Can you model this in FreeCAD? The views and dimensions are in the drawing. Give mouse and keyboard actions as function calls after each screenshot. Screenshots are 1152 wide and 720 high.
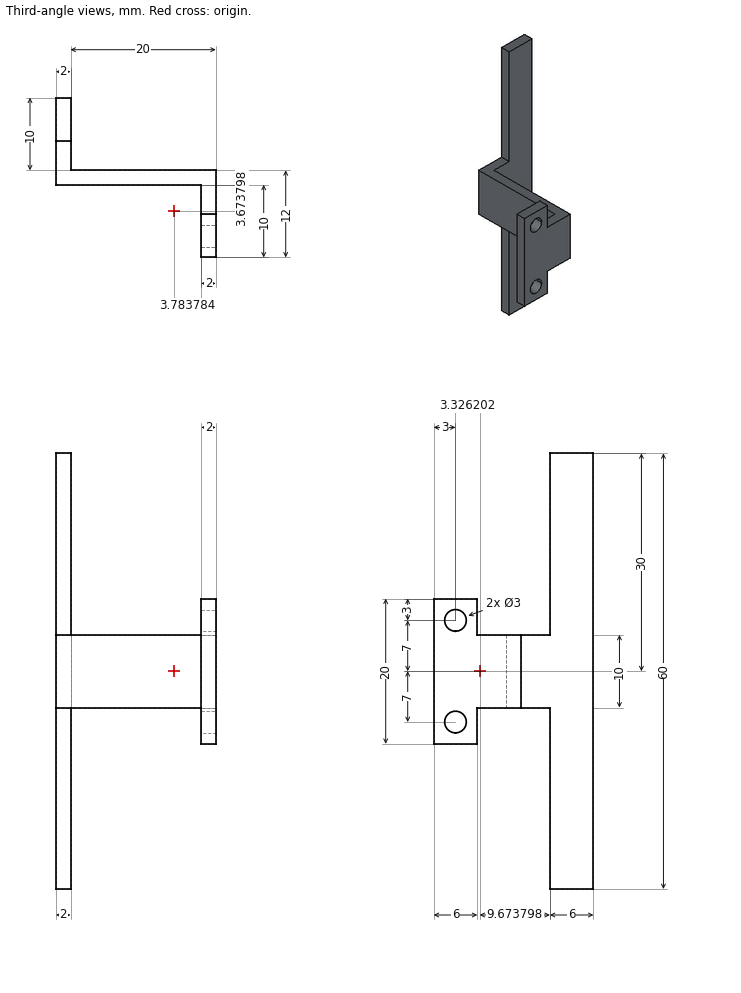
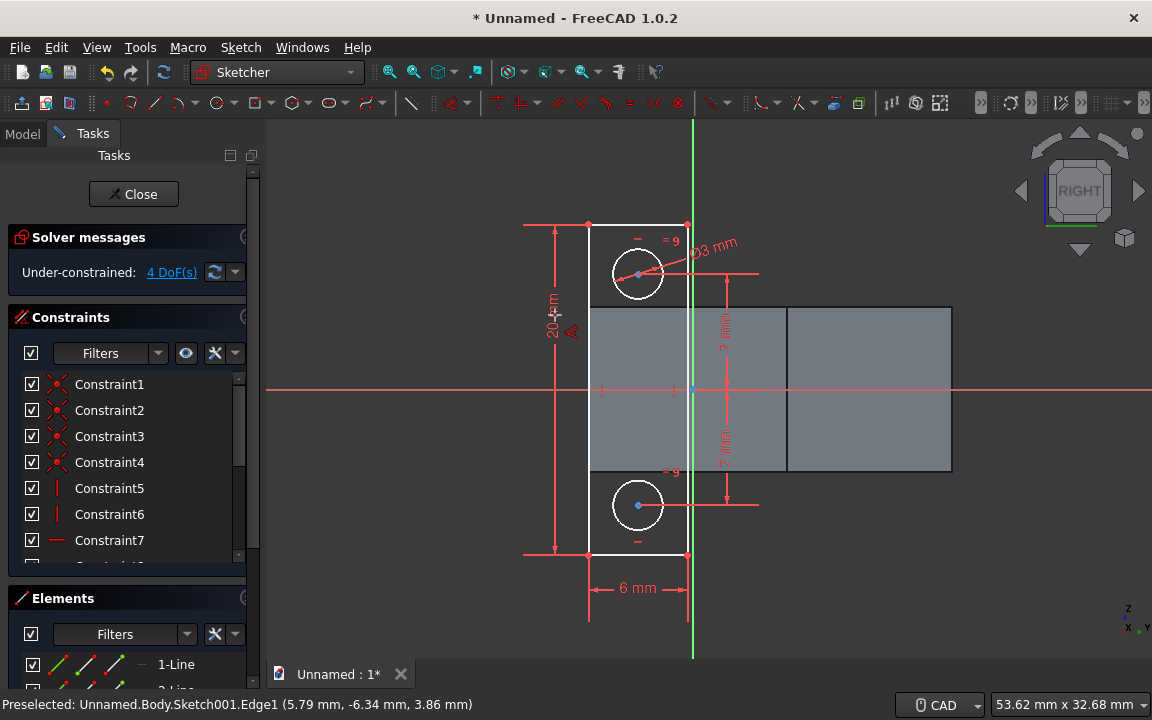
click(589, 225)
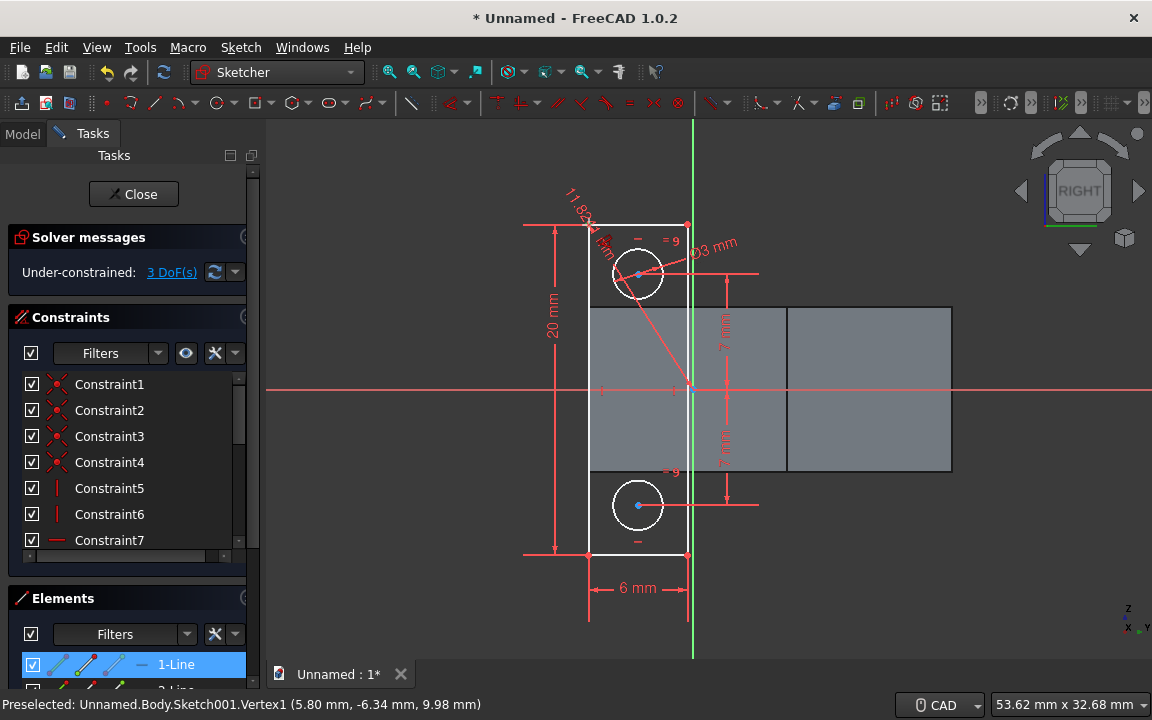
click(638, 274)
click(613, 191)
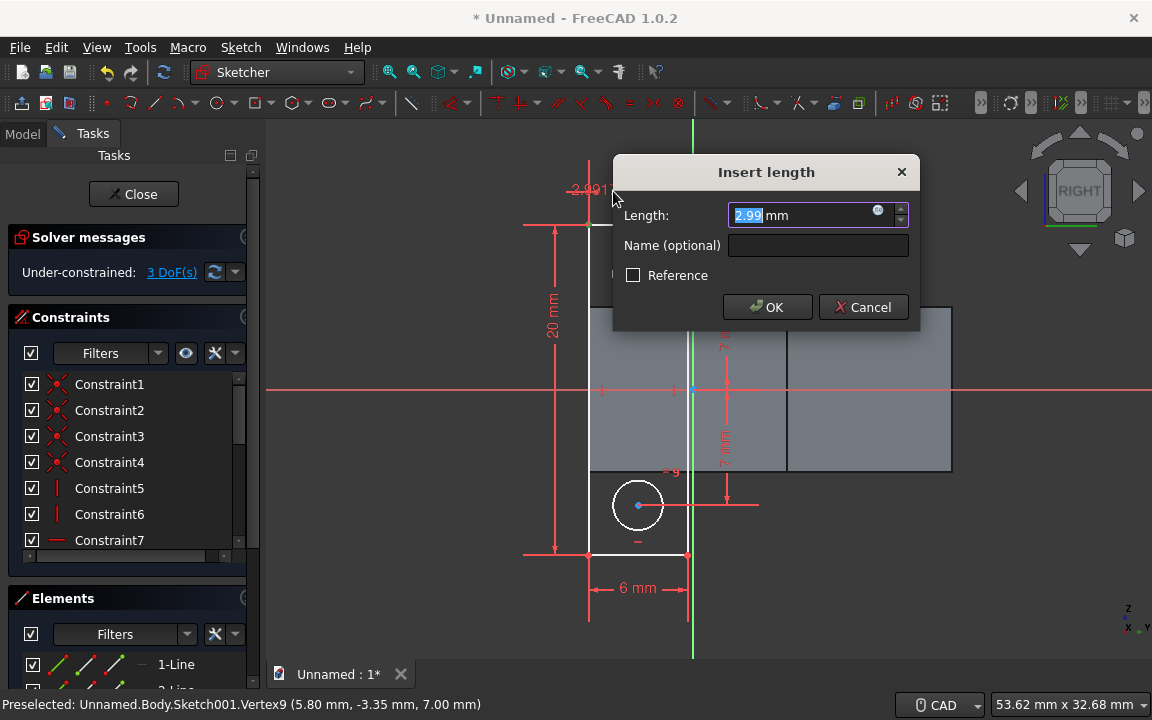
text(3)
key(Return)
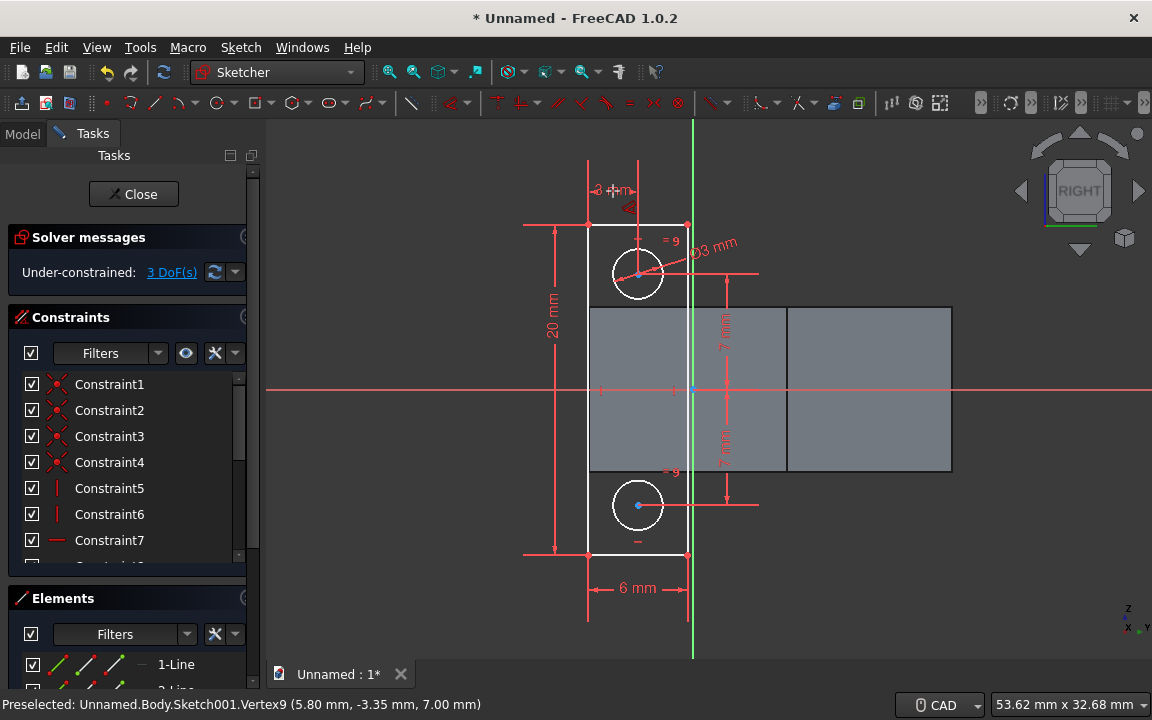
click(588, 225)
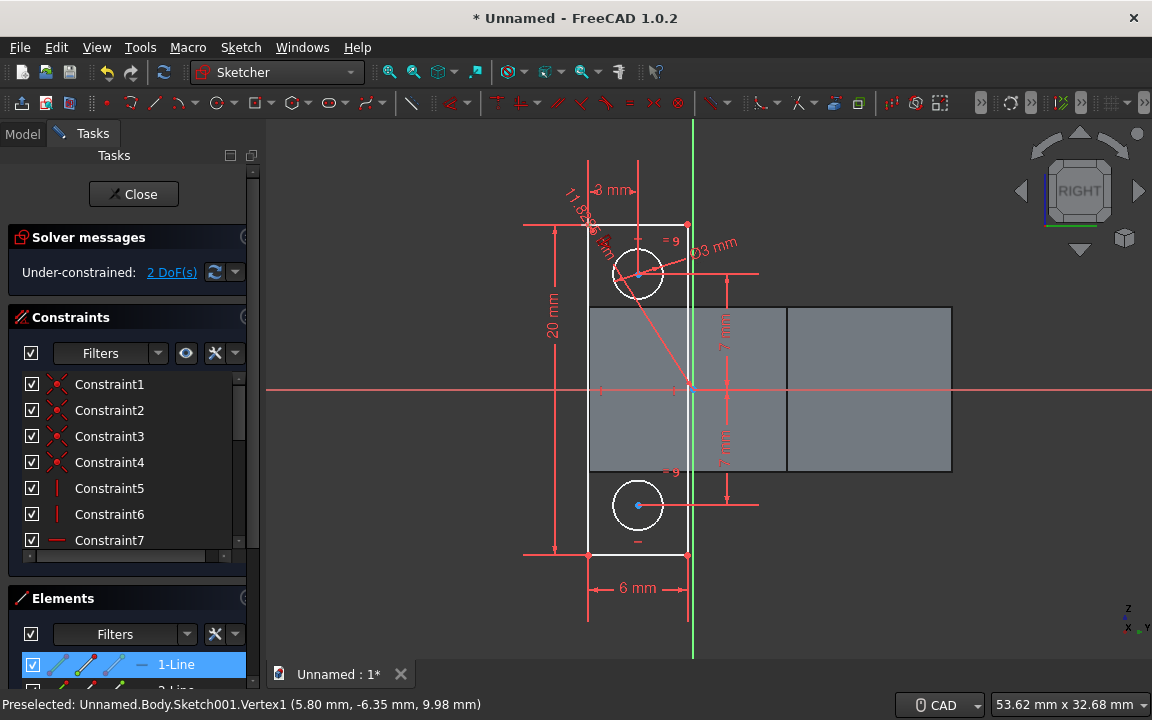
click(638, 274)
click(554, 249)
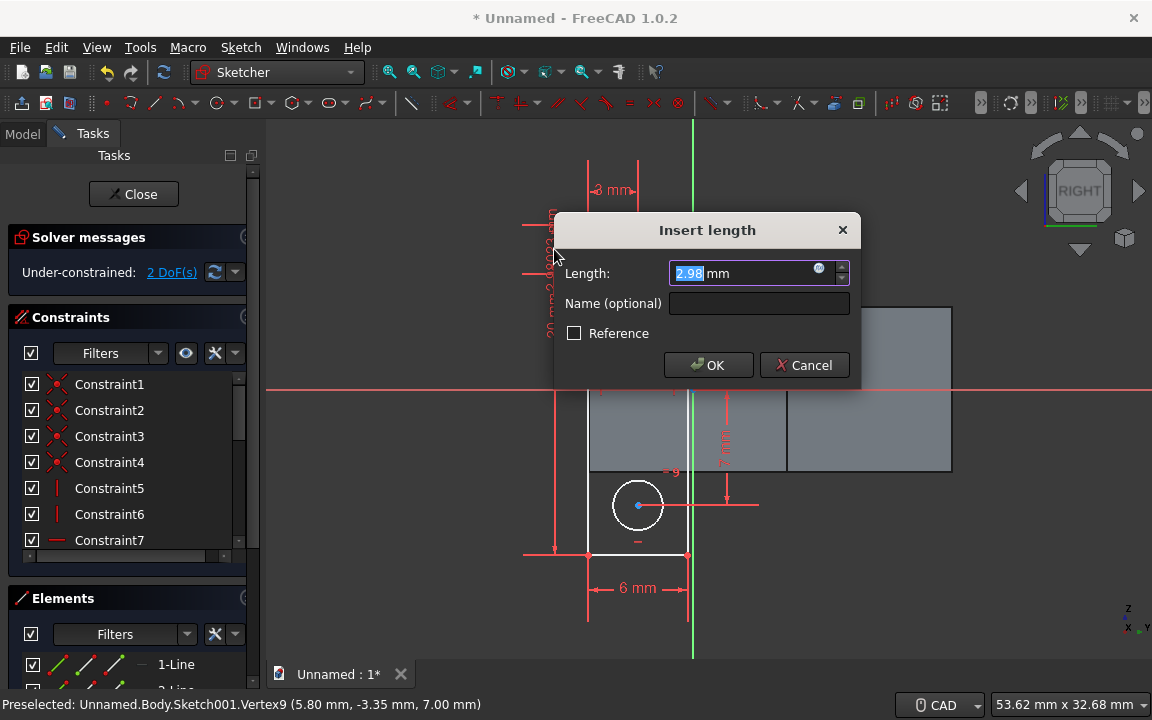
text(3)
key(Return)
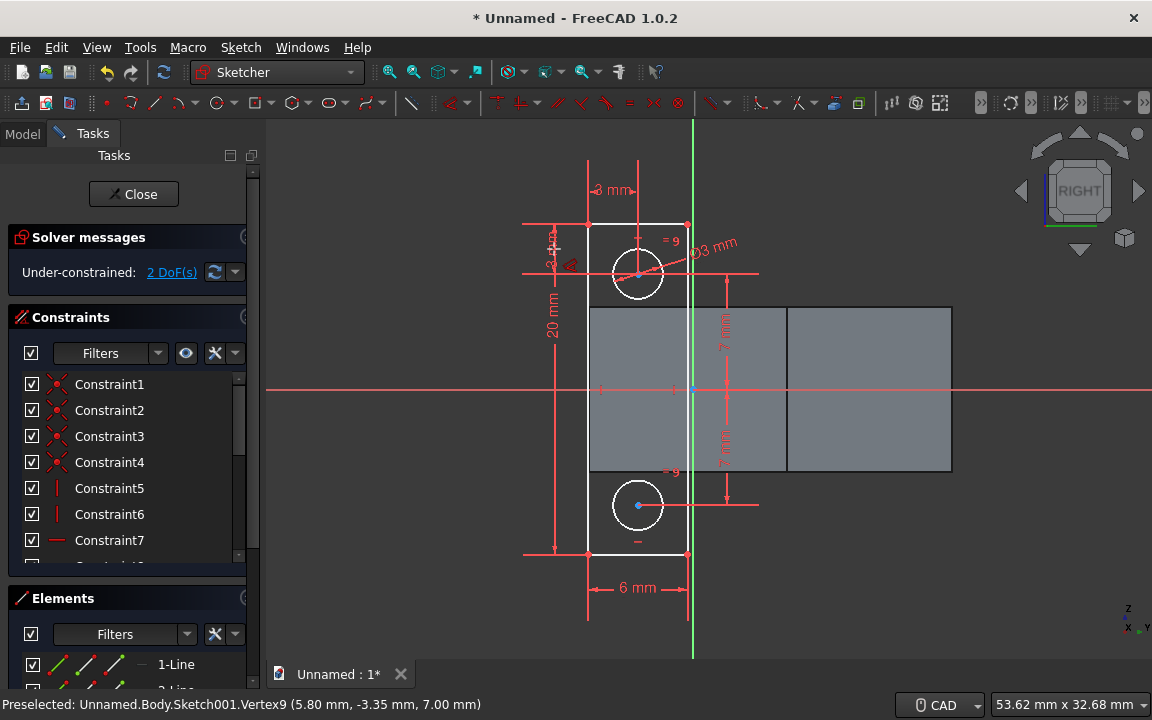
click(588, 555)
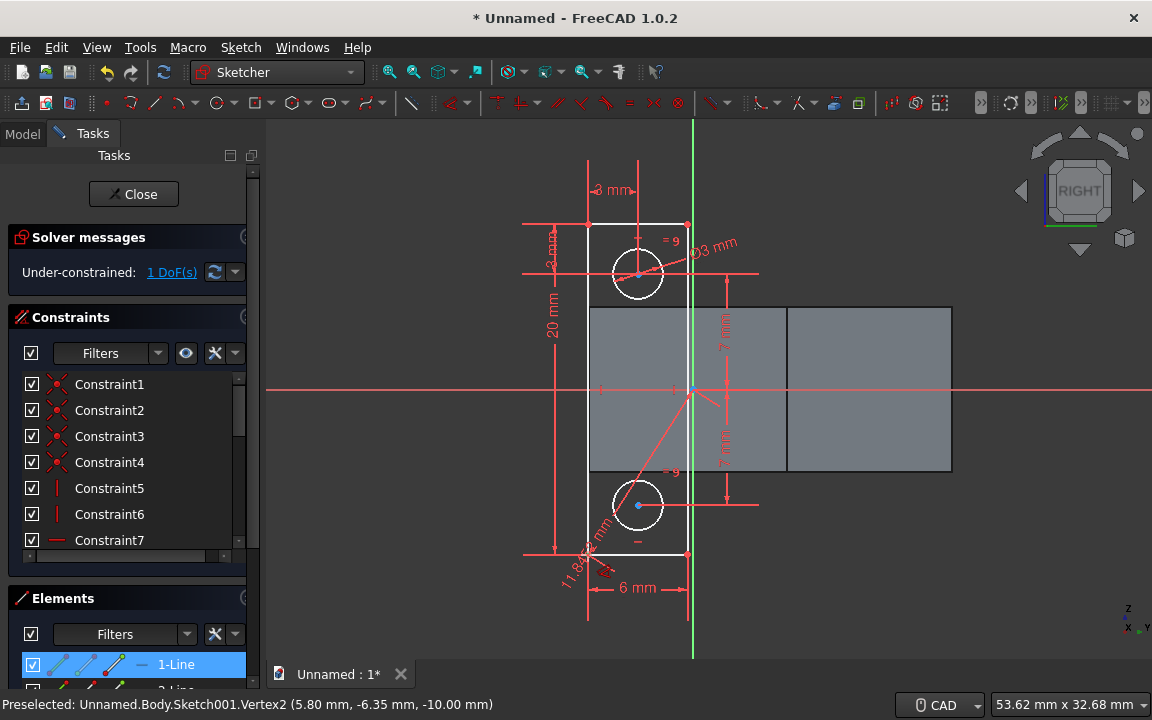
click(638, 505)
click(613, 471)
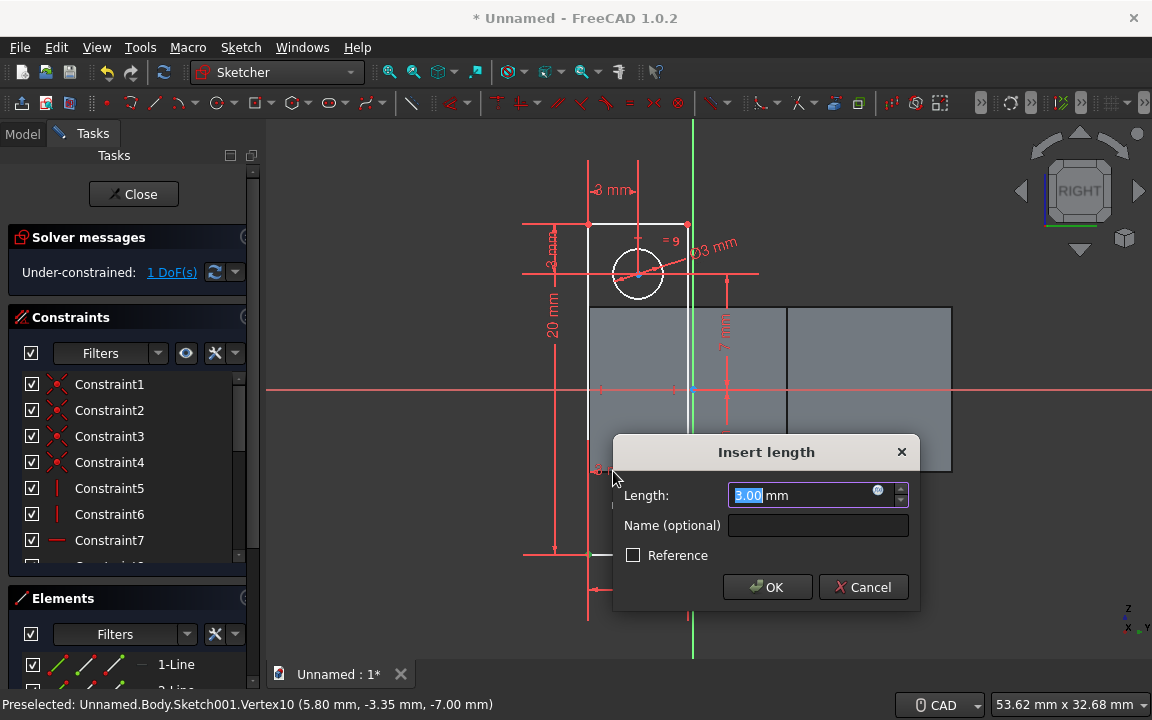
text(3)
key(Return)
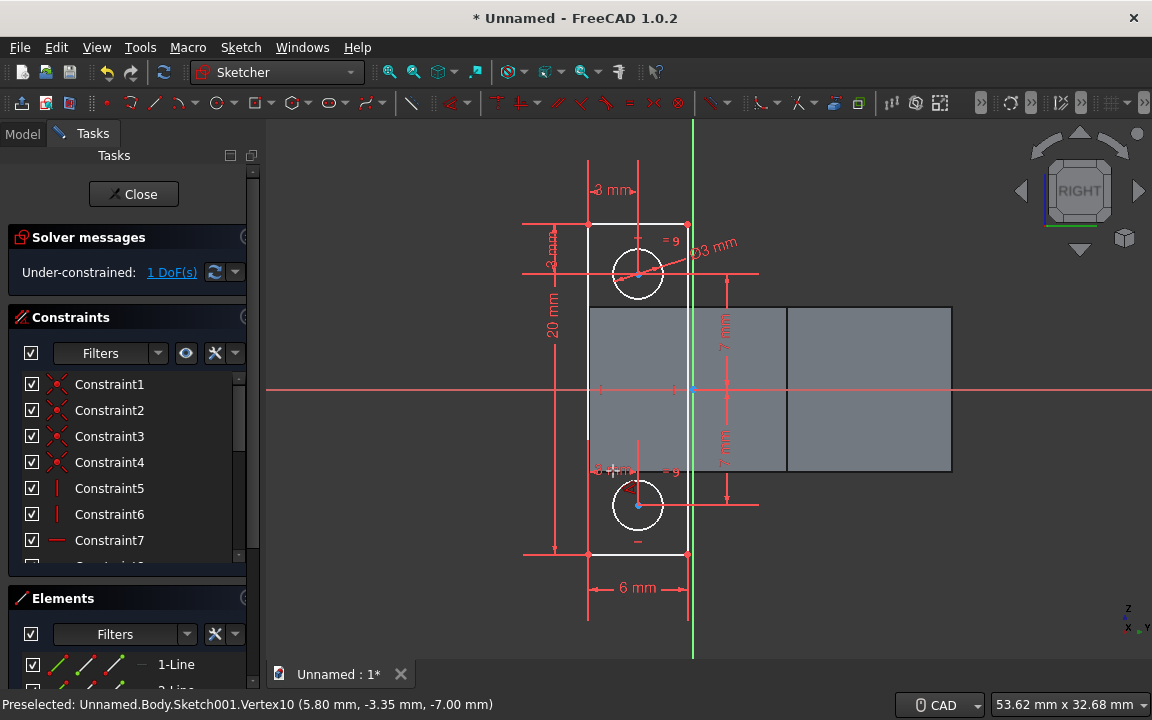
click(638, 274)
click(666, 424)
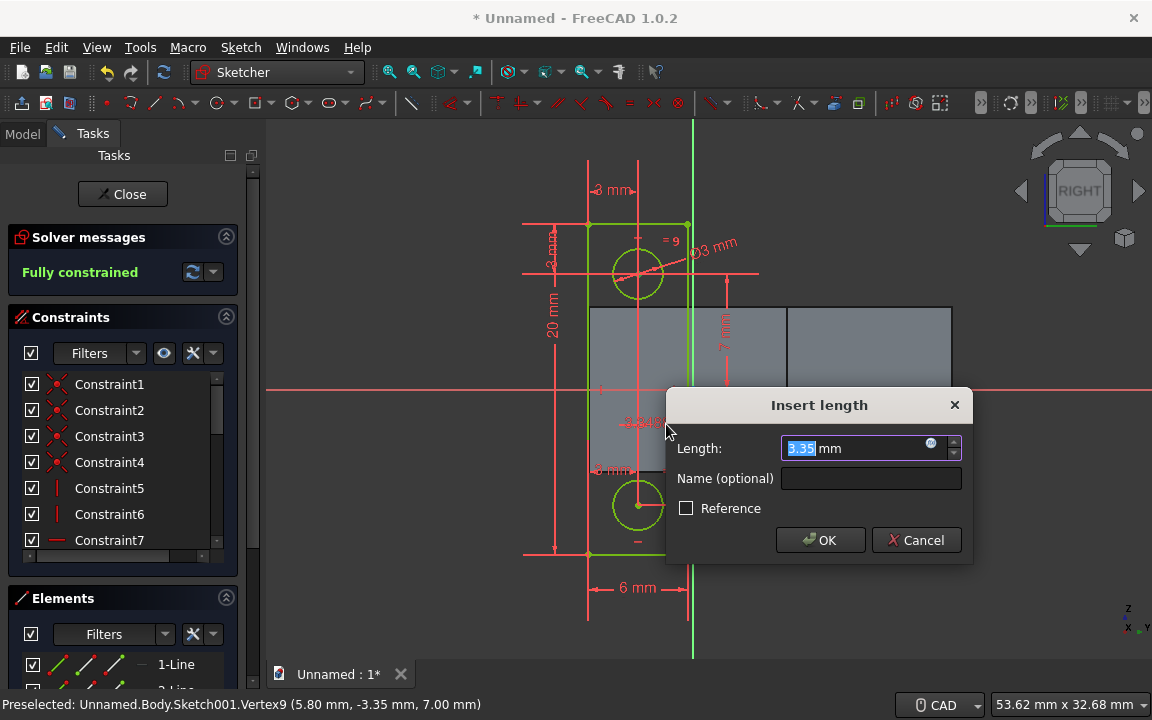
text(3.326202)
key(Return)
key(Escape)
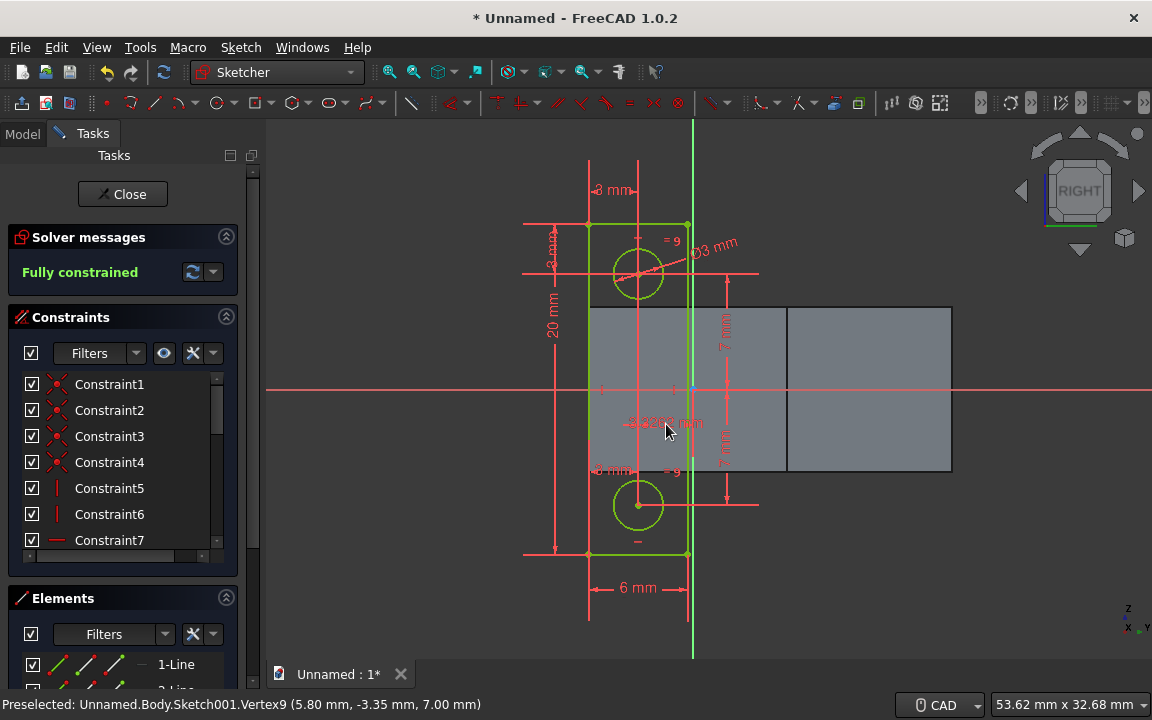
click(123, 194)